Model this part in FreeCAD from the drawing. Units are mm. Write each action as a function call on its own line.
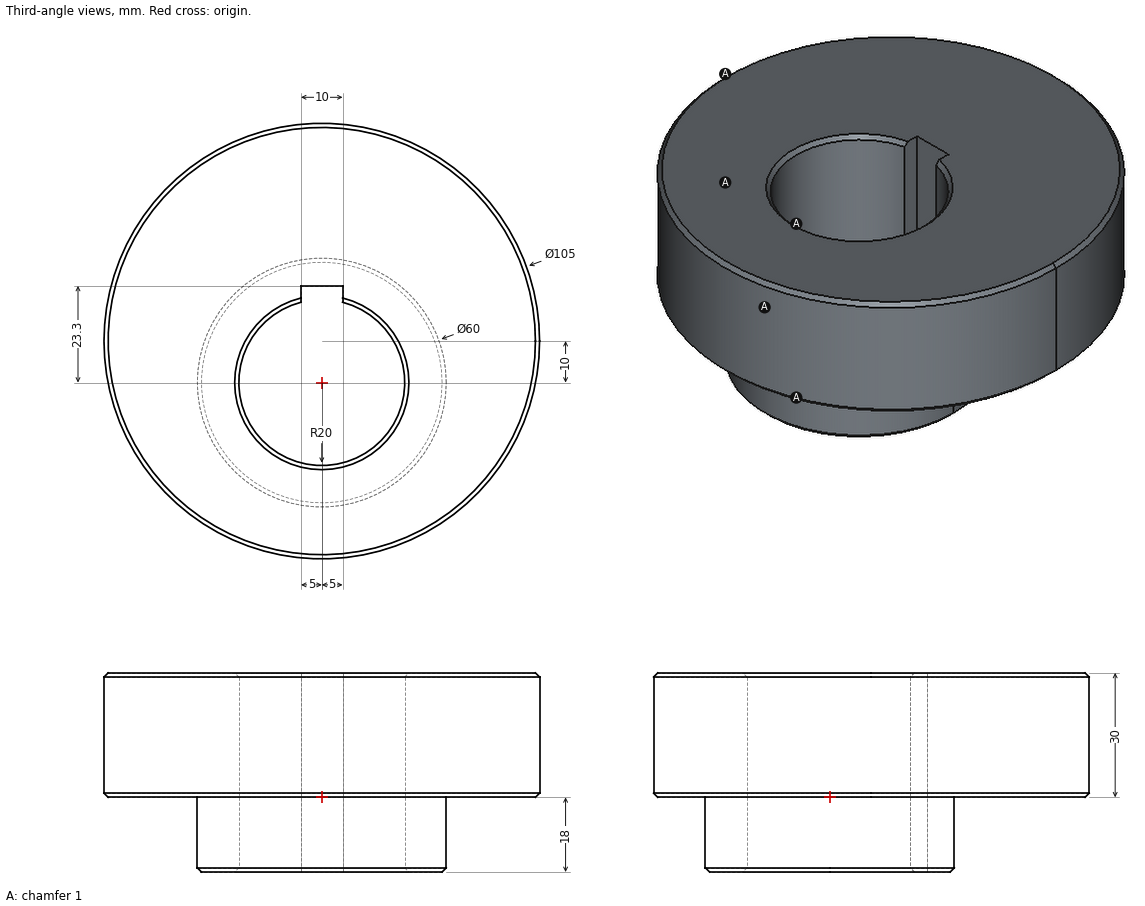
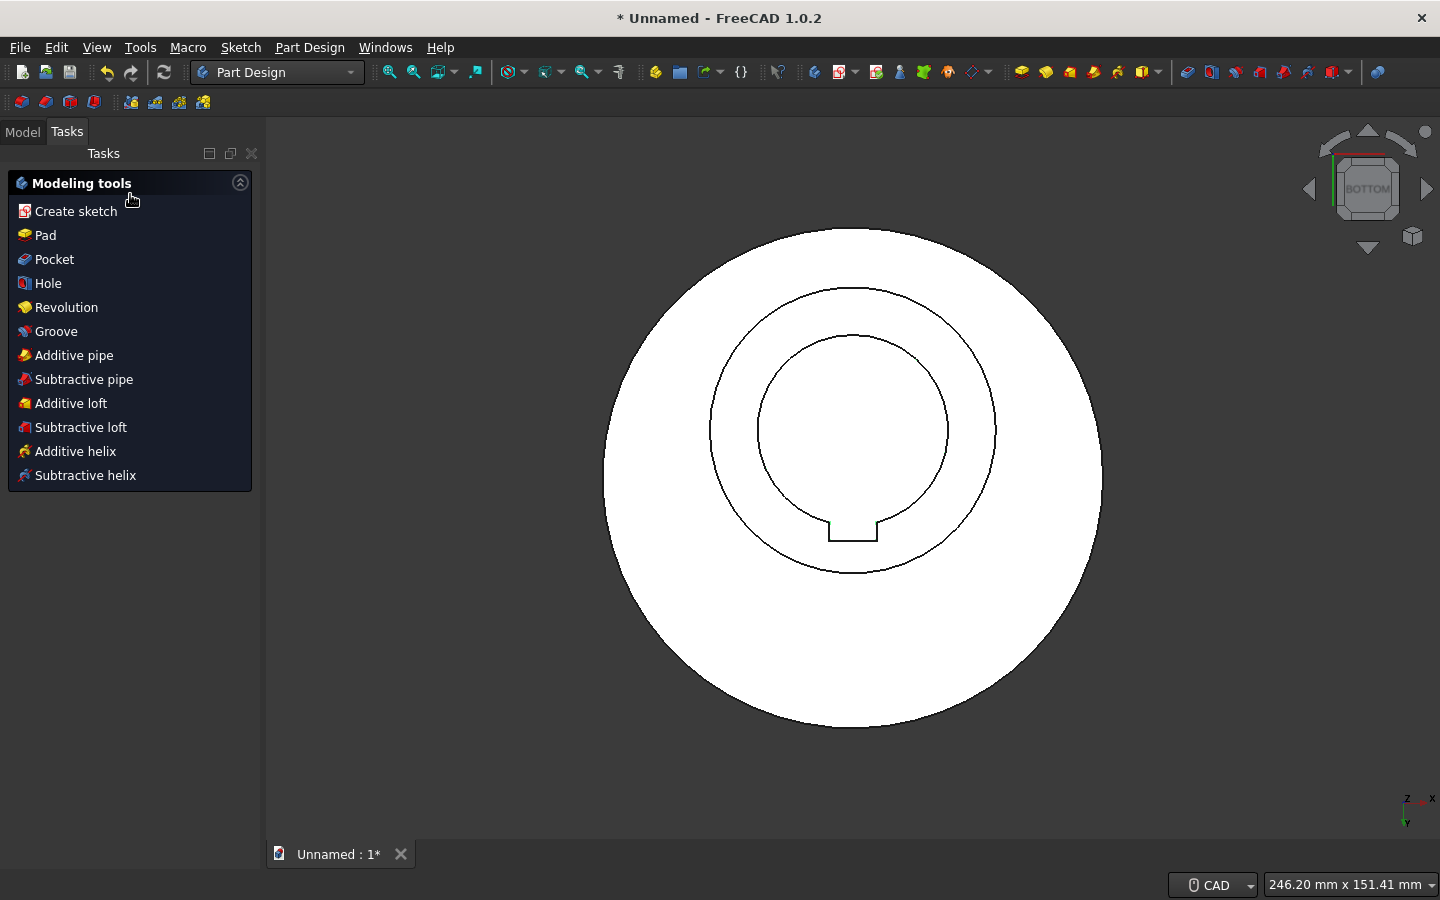
click(1188, 72)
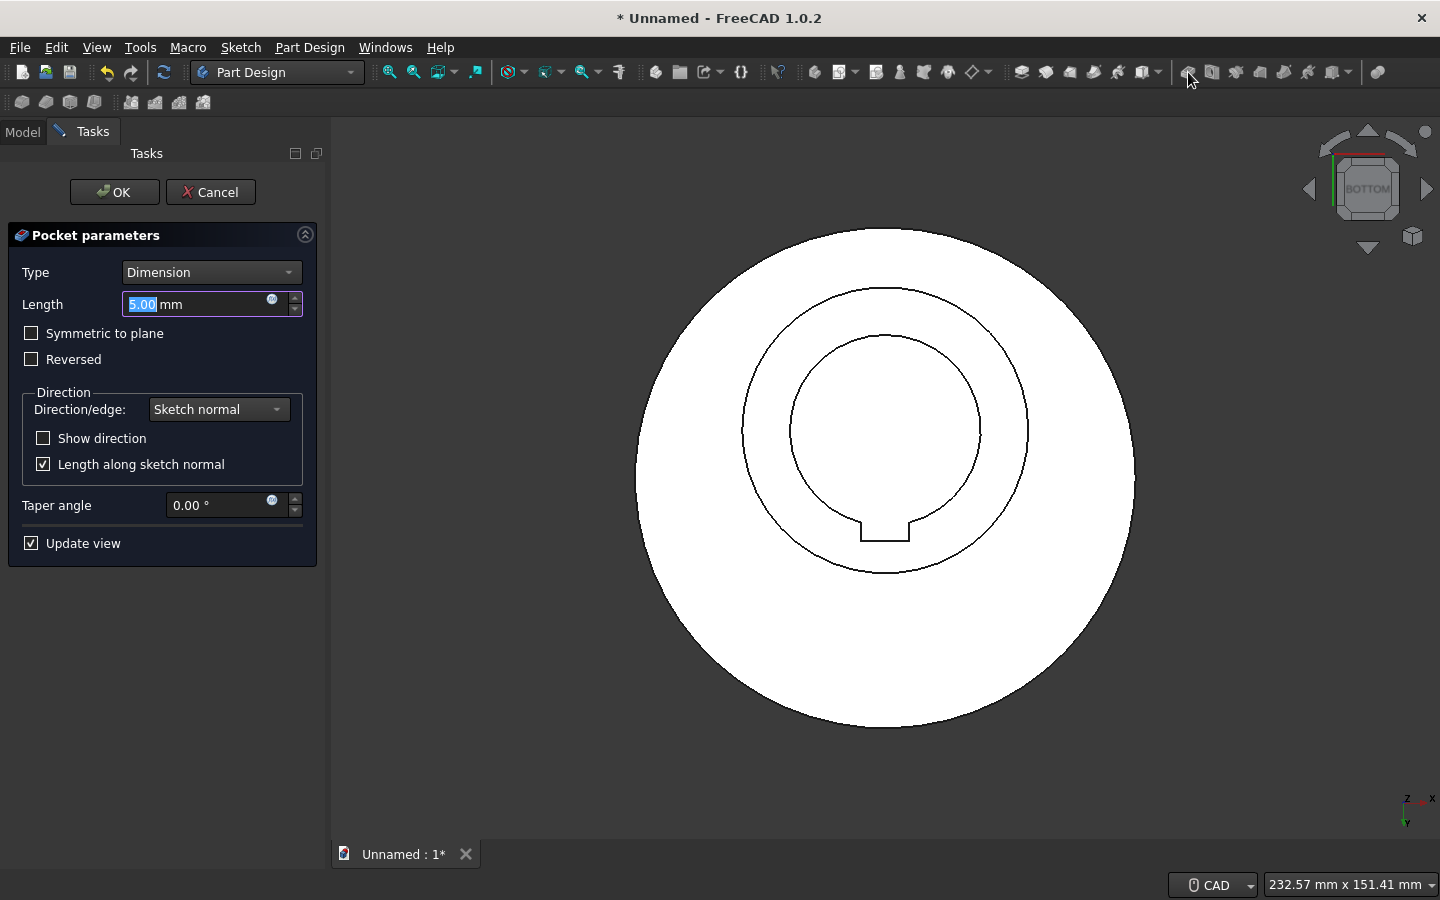
click(212, 272)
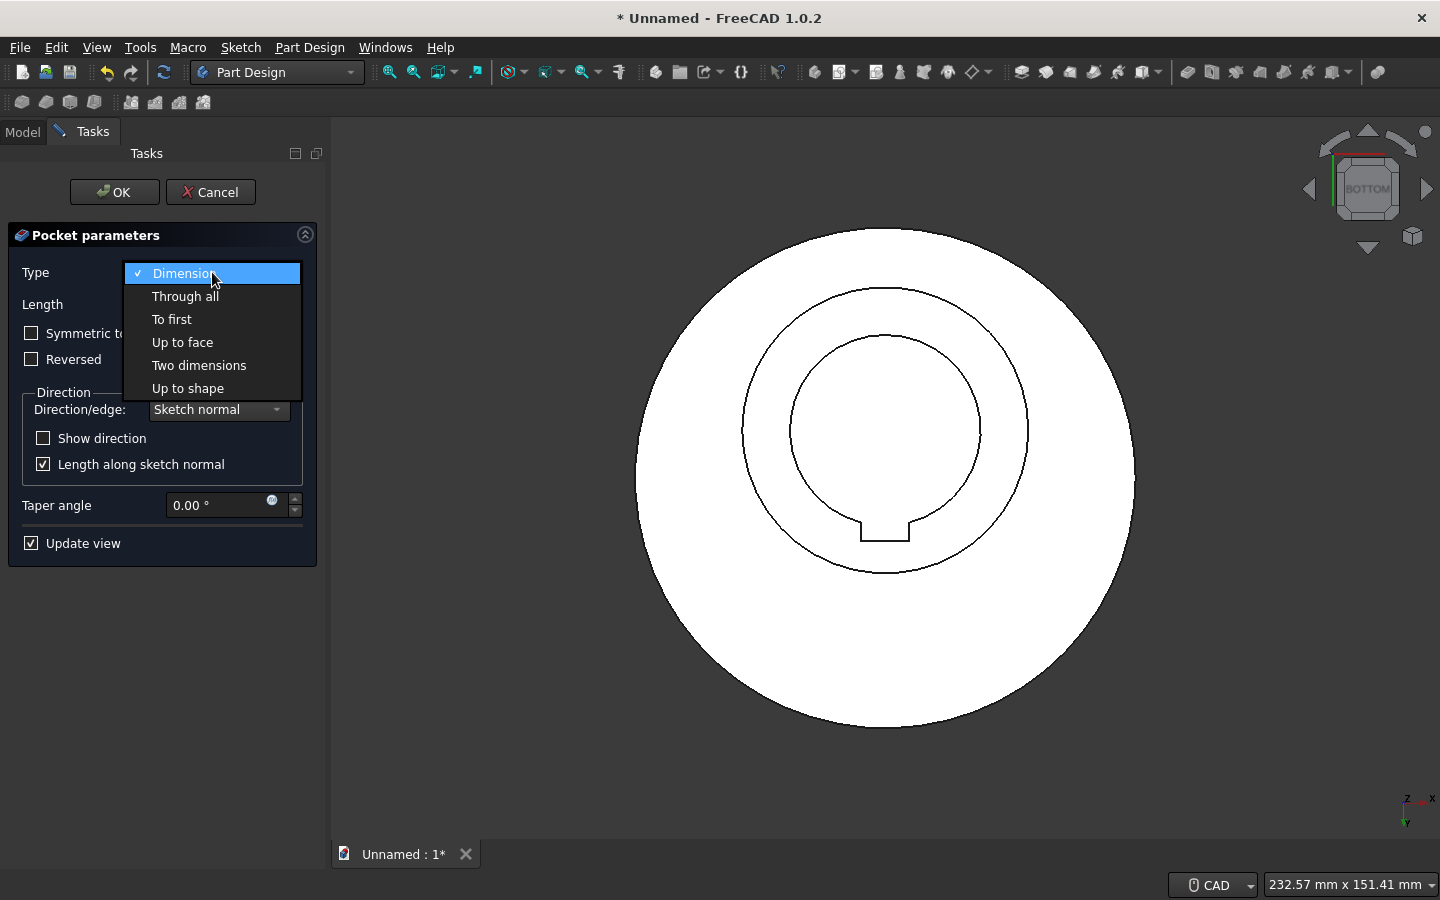
click(212, 296)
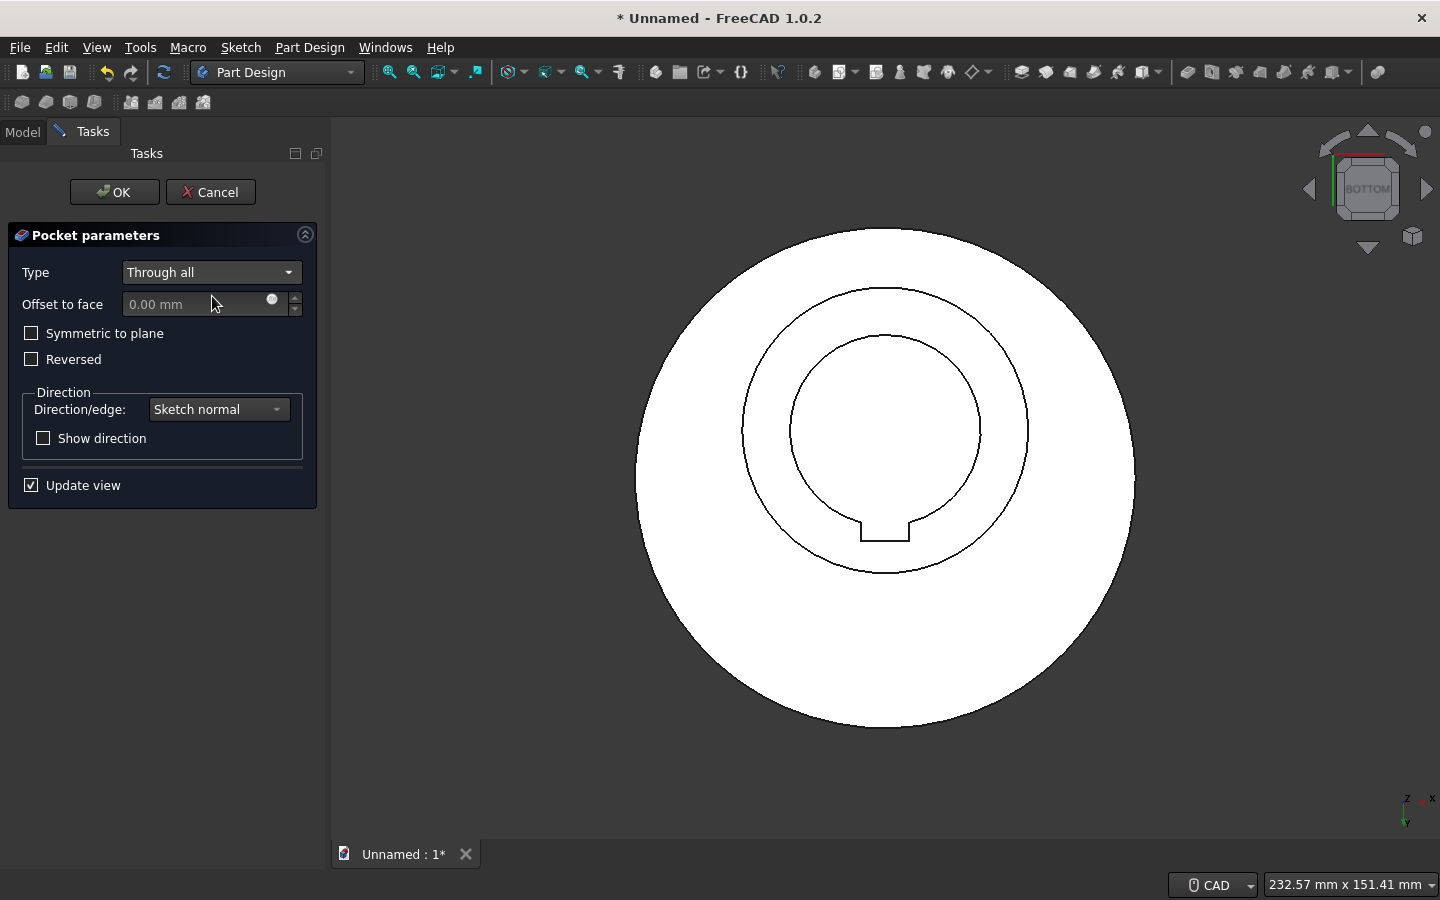
click(30, 359)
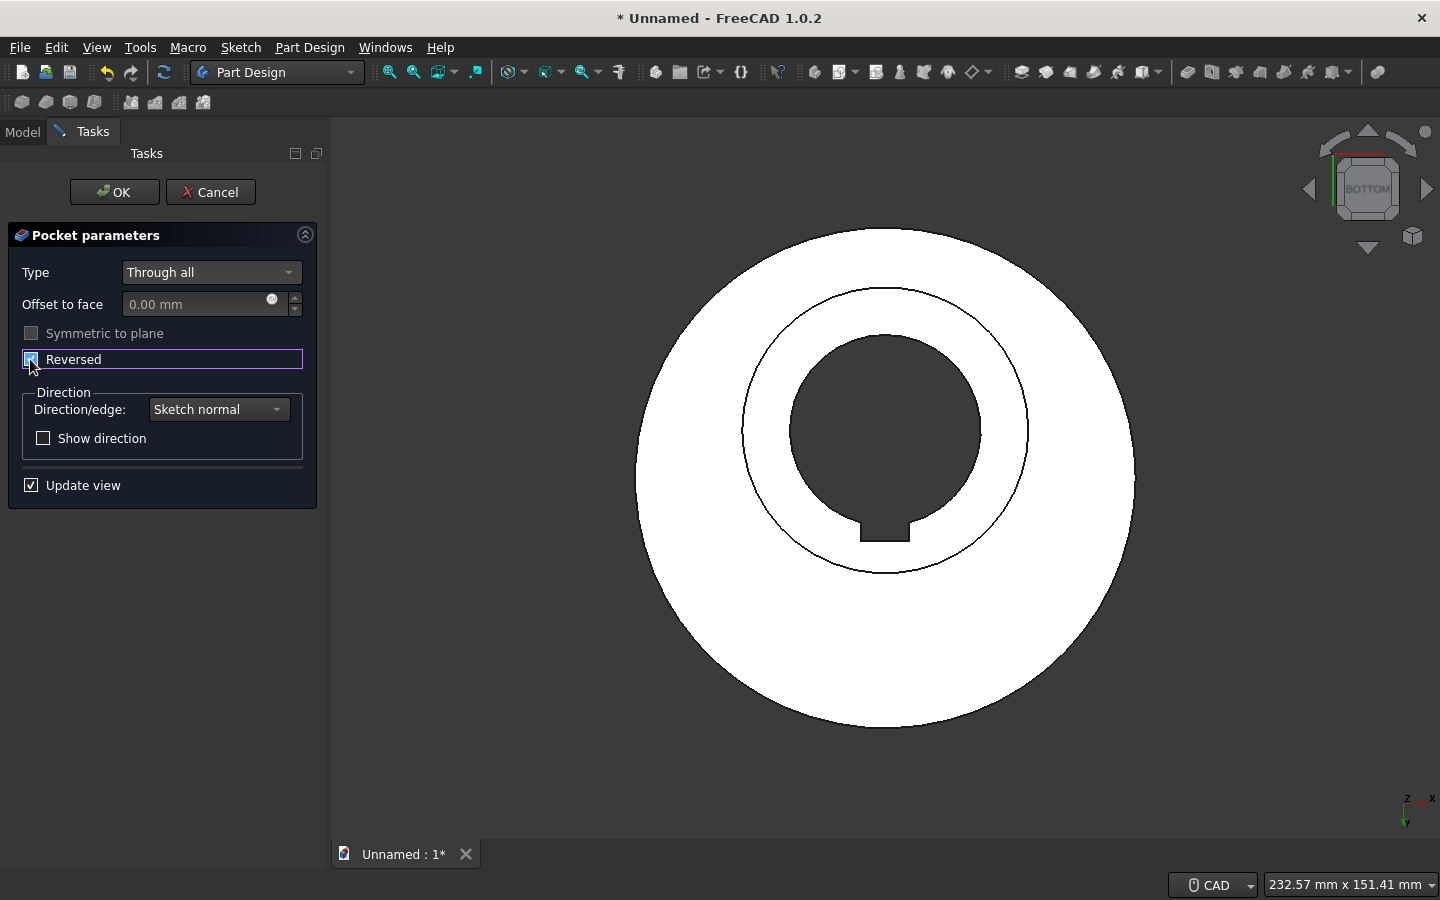
click(115, 192)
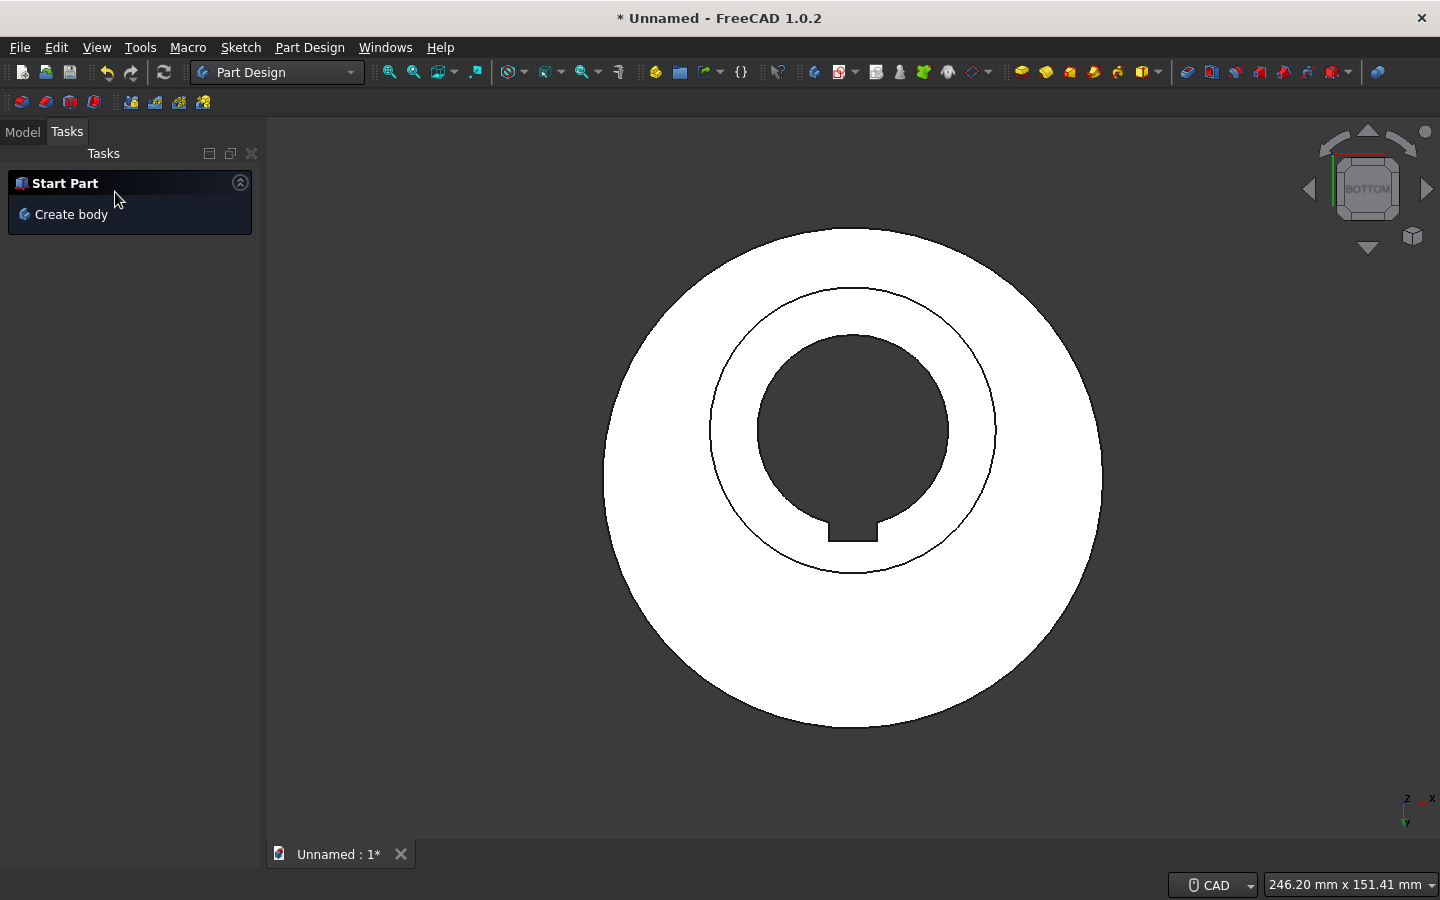
click(602, 477)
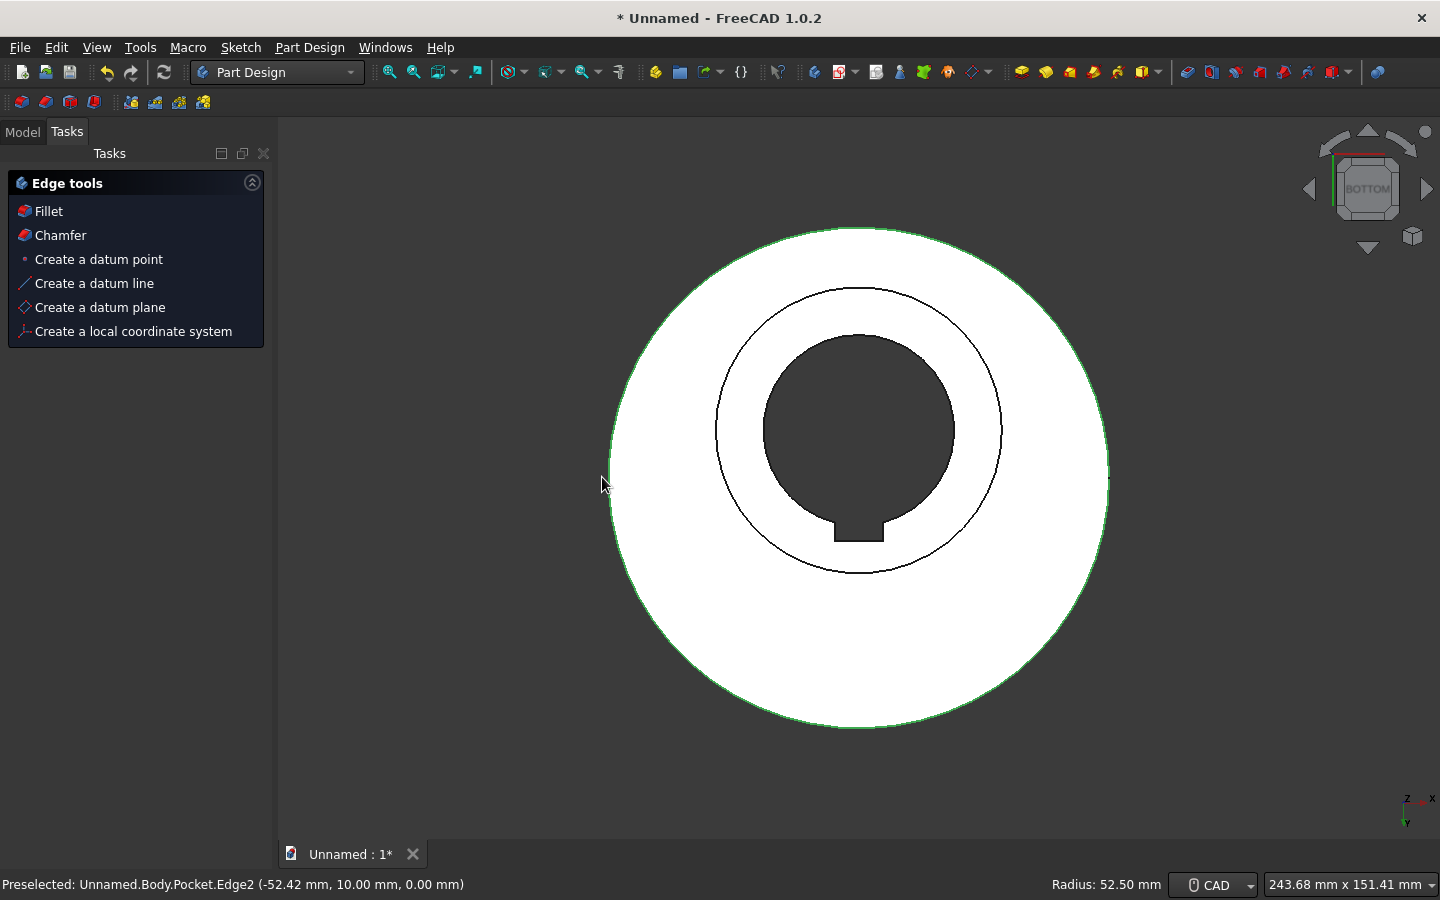
click(716, 429, ctrl)